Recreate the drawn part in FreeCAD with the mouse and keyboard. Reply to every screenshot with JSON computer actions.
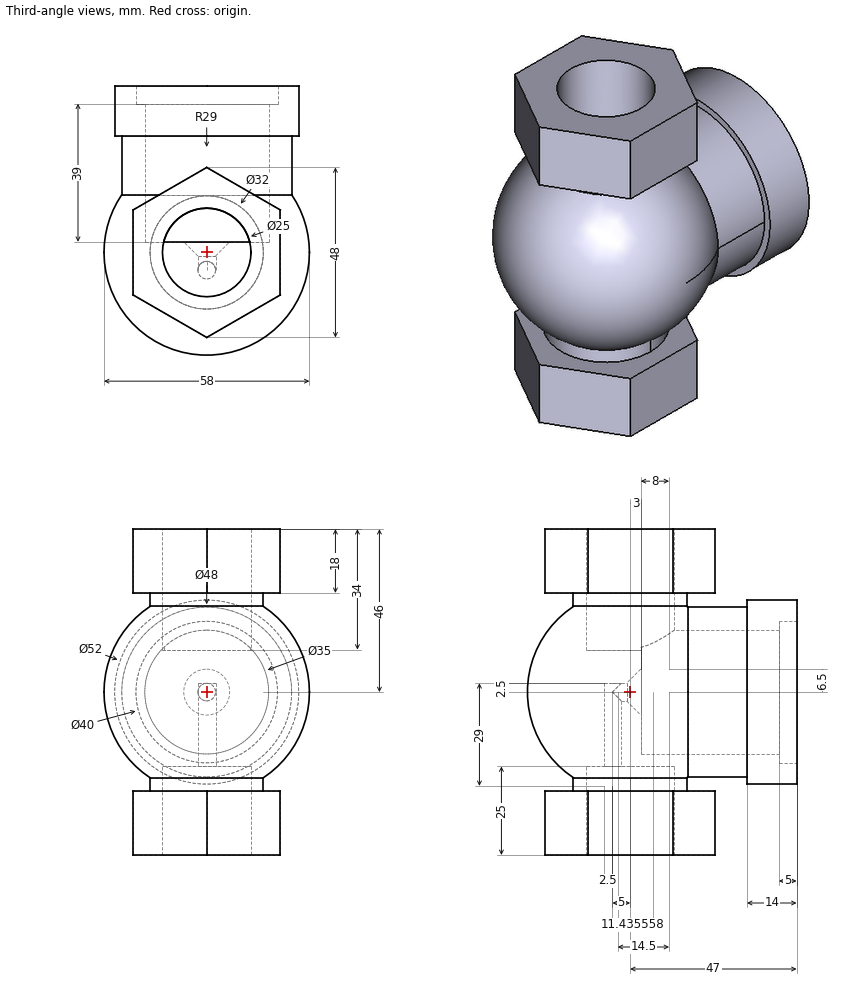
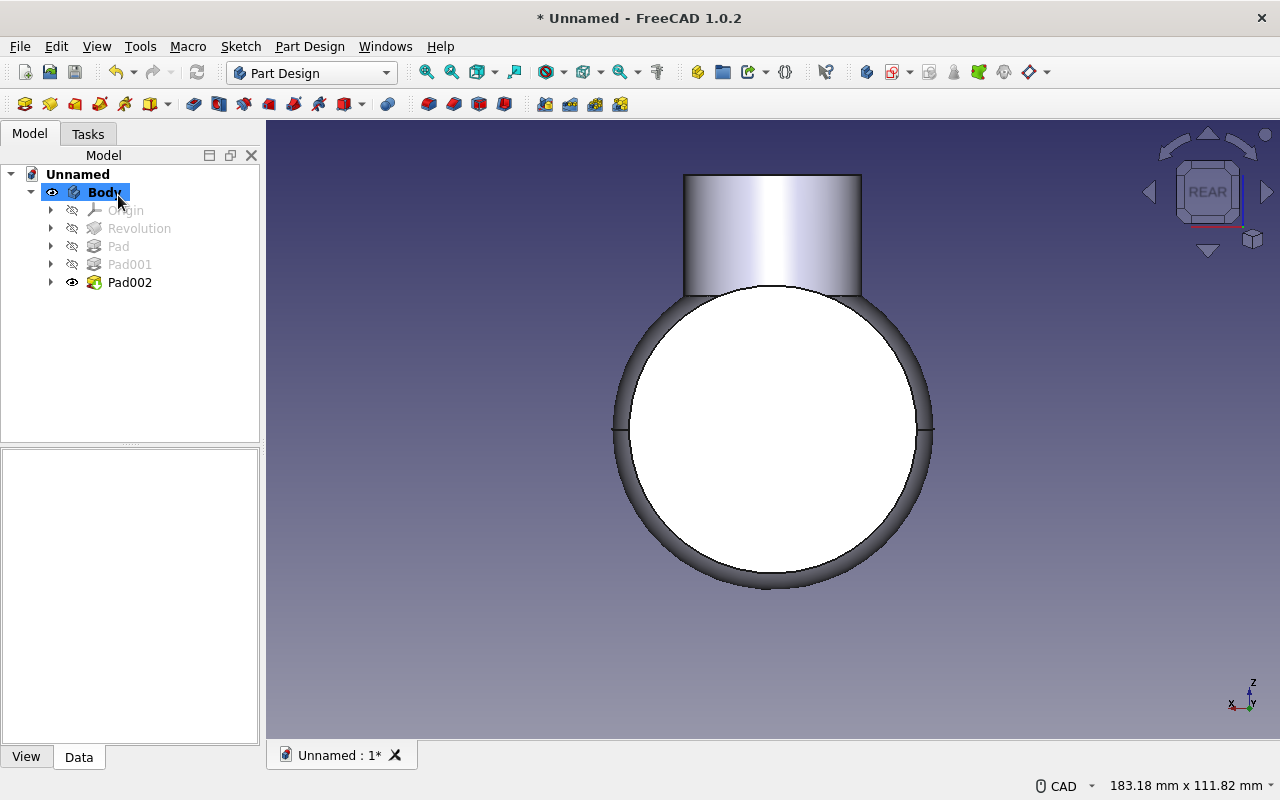
{"action": "left_click", "coordinate": [51, 210]}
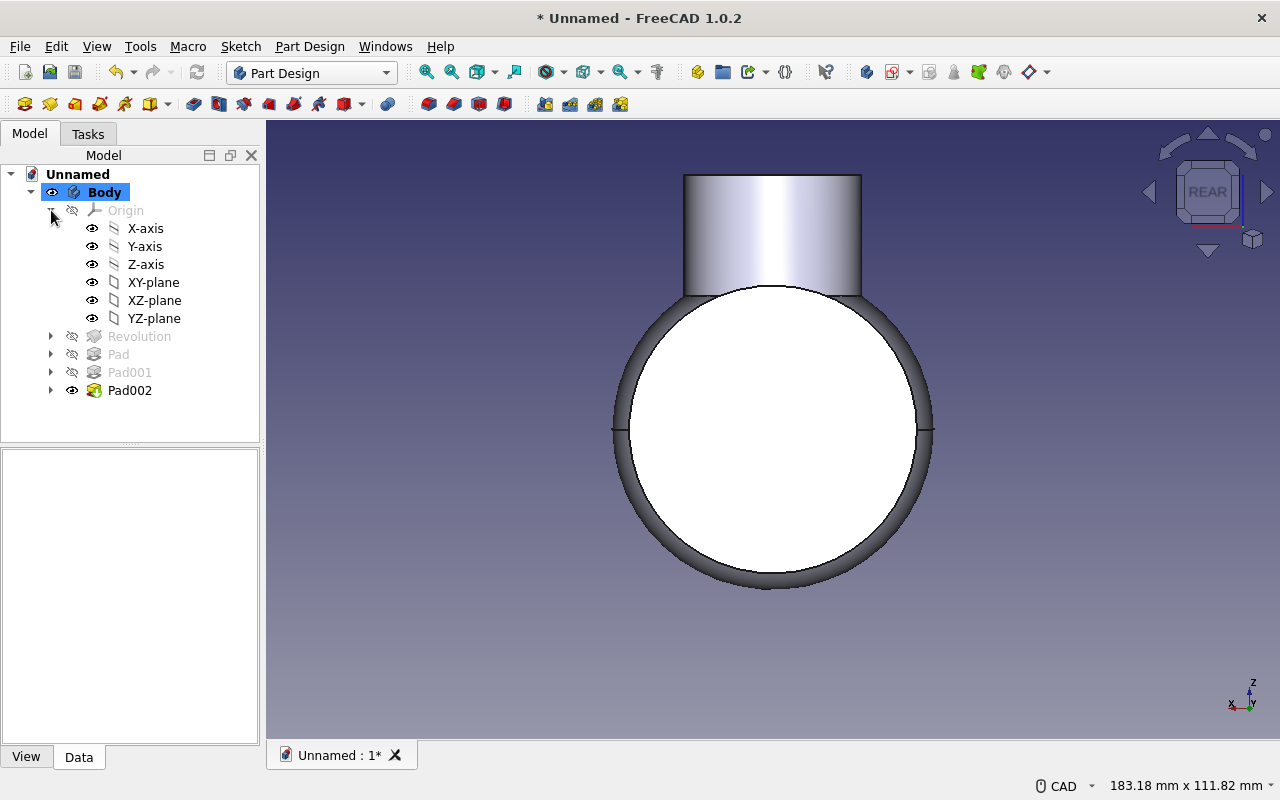
{"action": "left_click", "coordinate": [137, 282]}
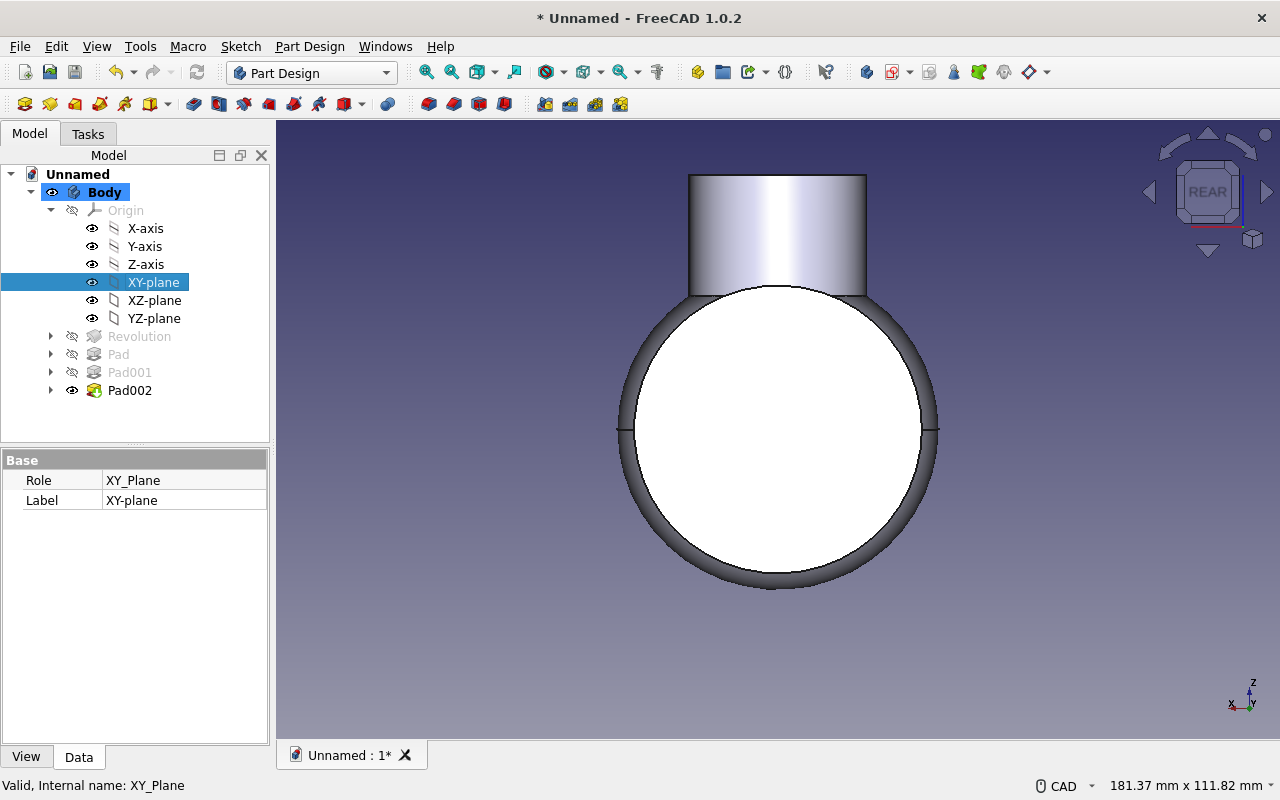
{"action": "left_click", "coordinate": [1028, 72]}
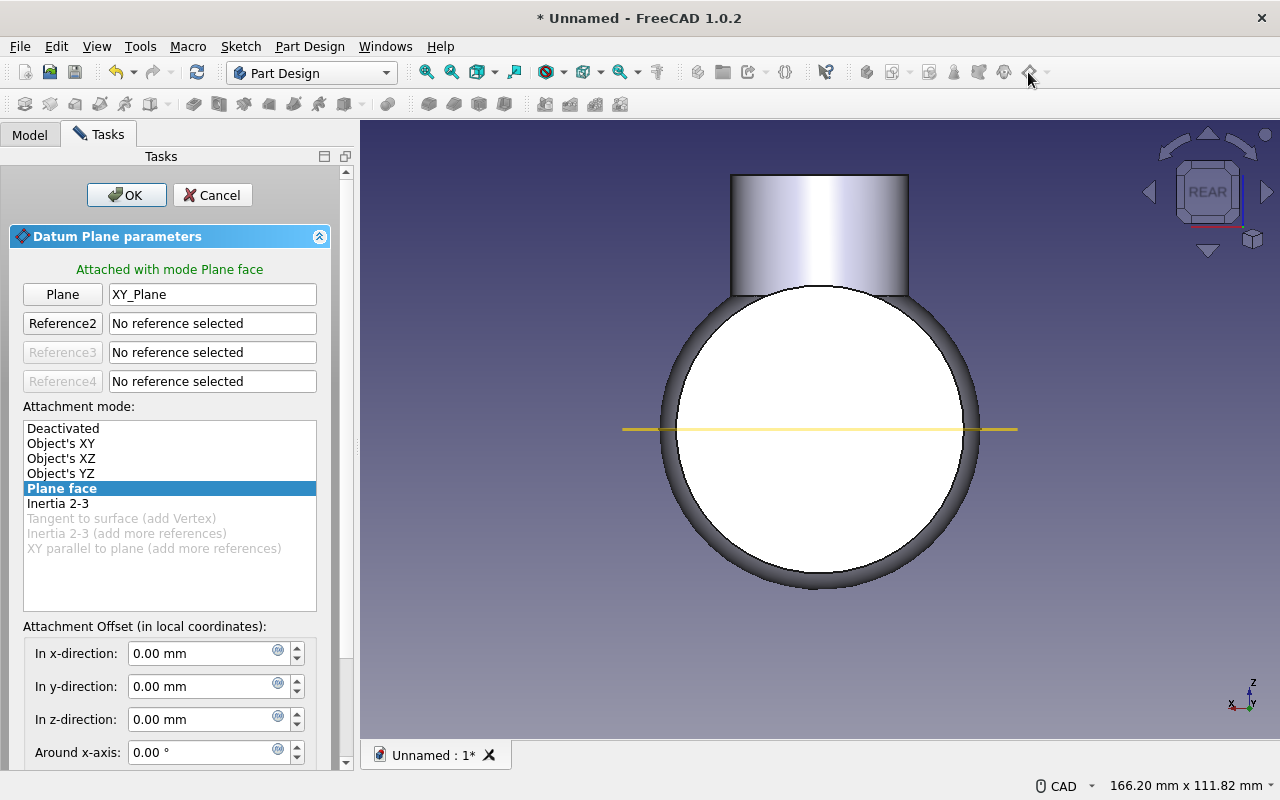
{"action": "triple_click", "coordinate": [210, 720]}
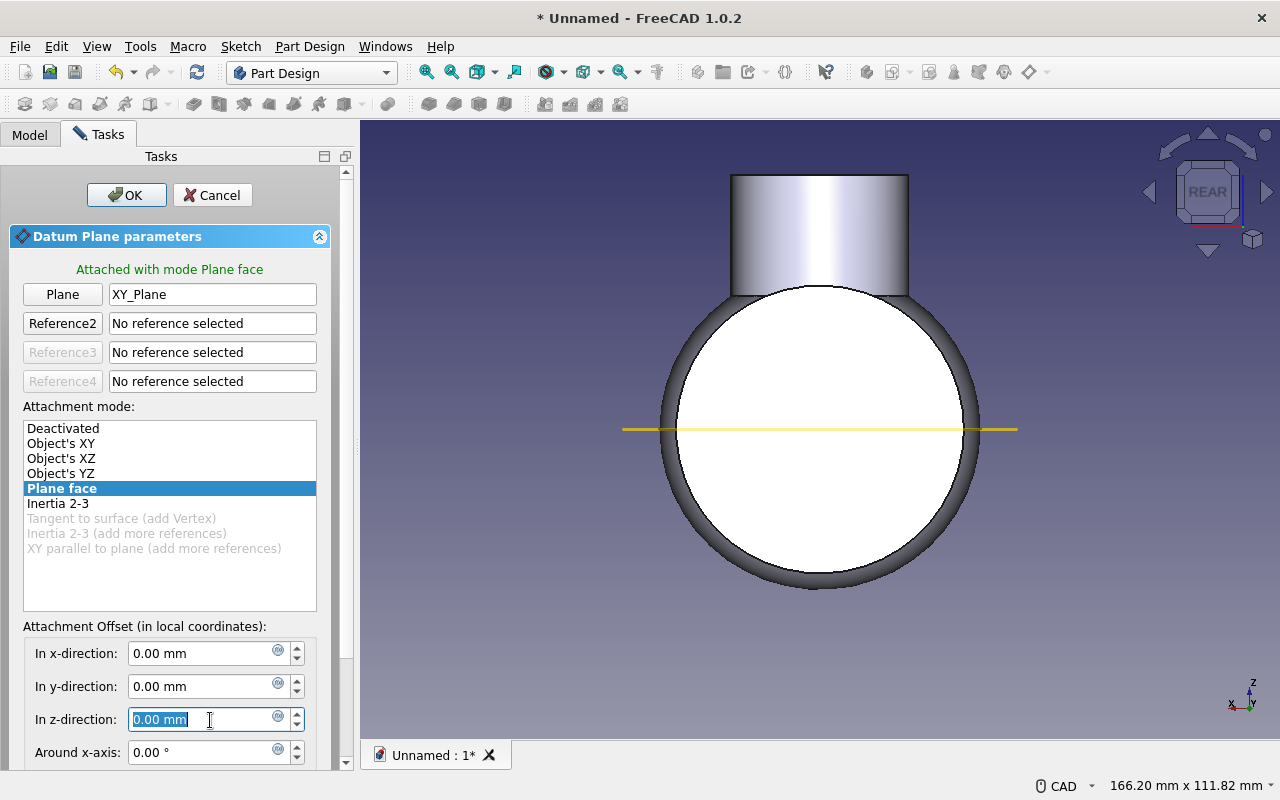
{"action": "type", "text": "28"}
{"action": "key", "text": "Tab"}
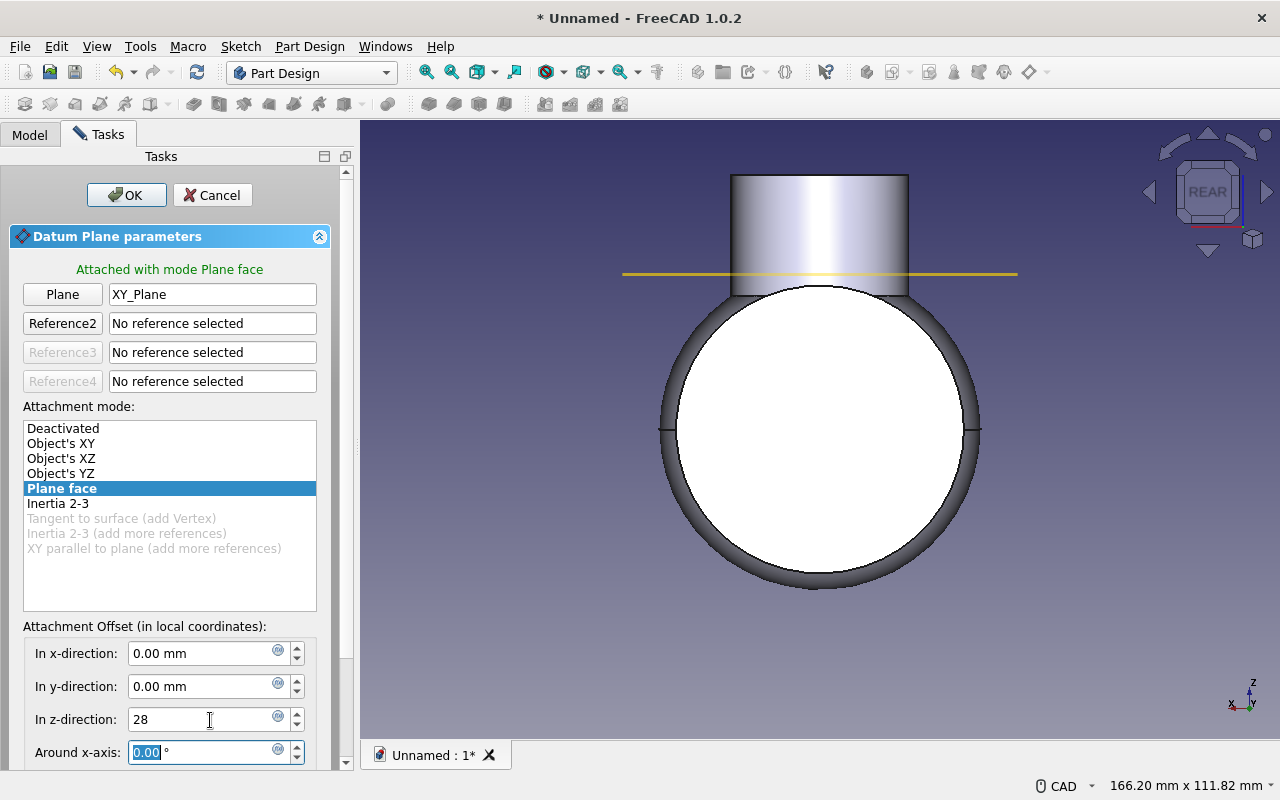
{"action": "left_click", "coordinate": [127, 195]}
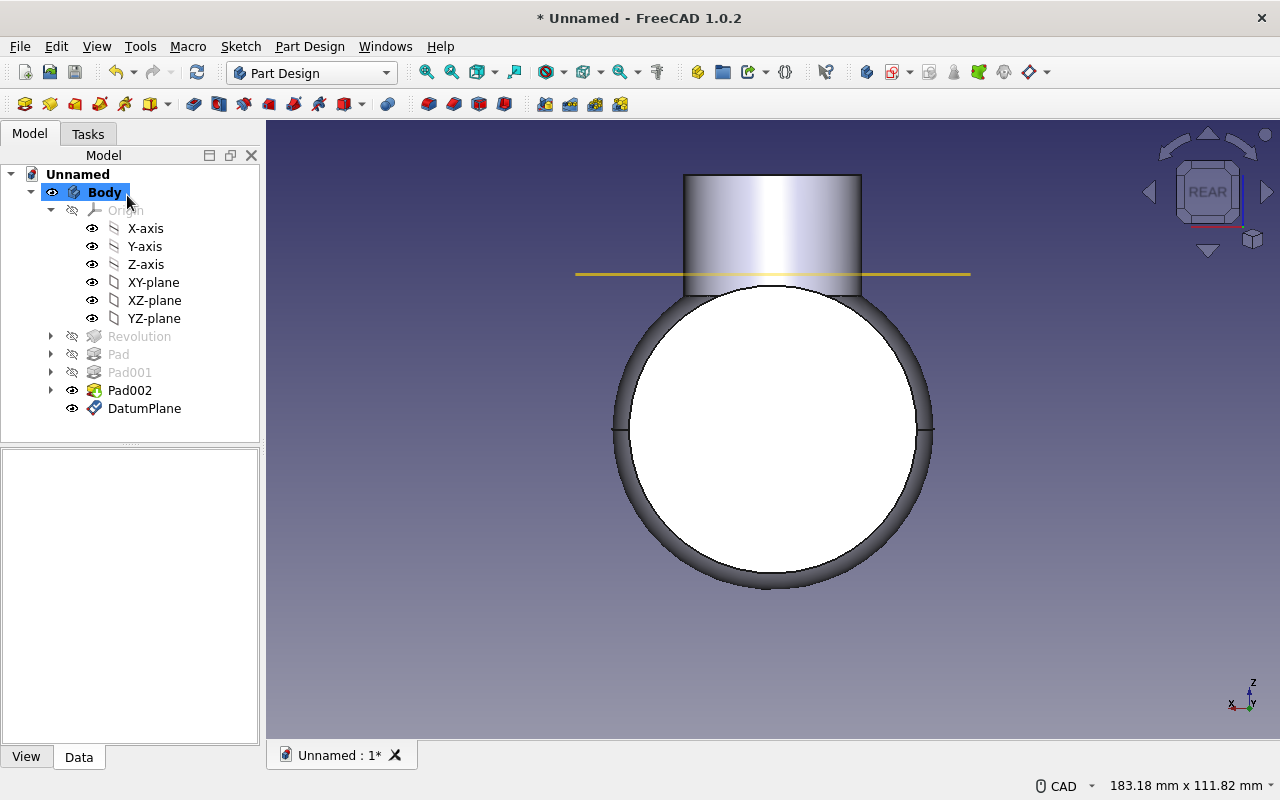
{"action": "left_click", "coordinate": [117, 408]}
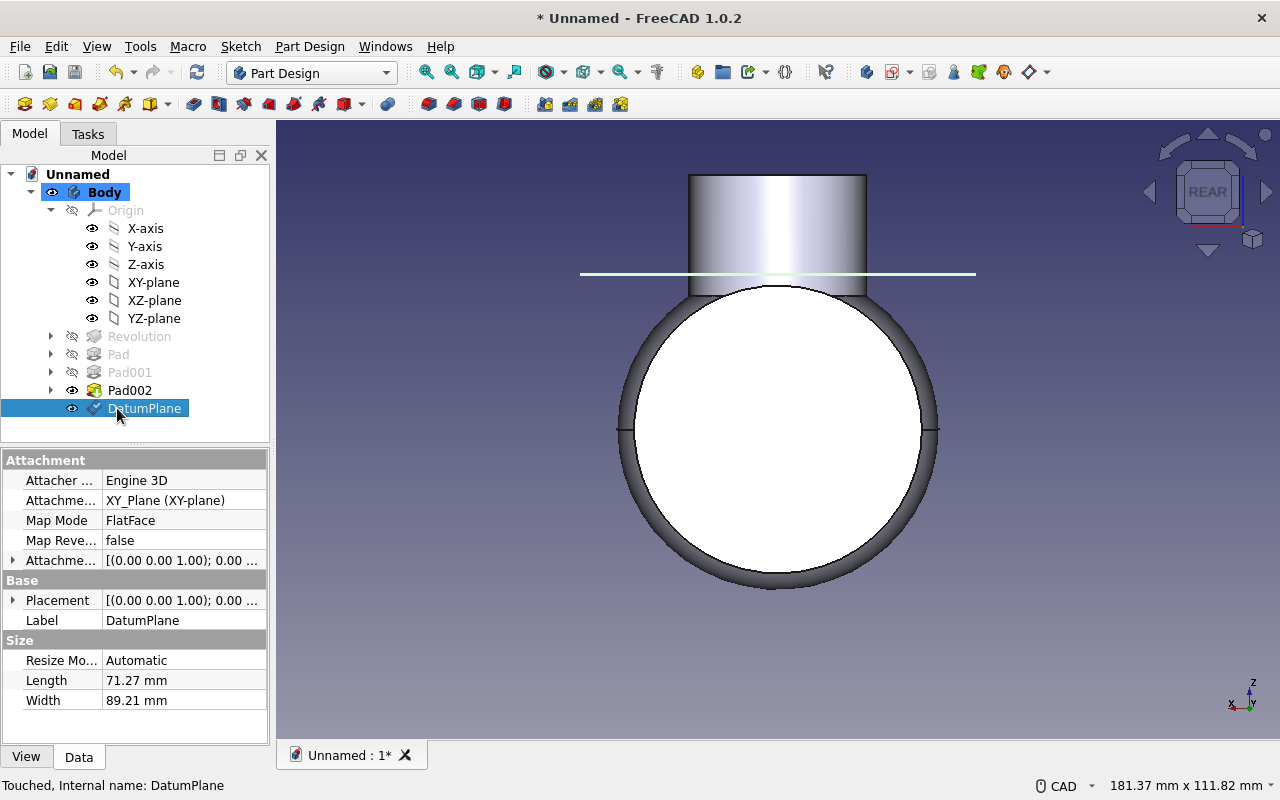
{"action": "left_click", "coordinate": [892, 72]}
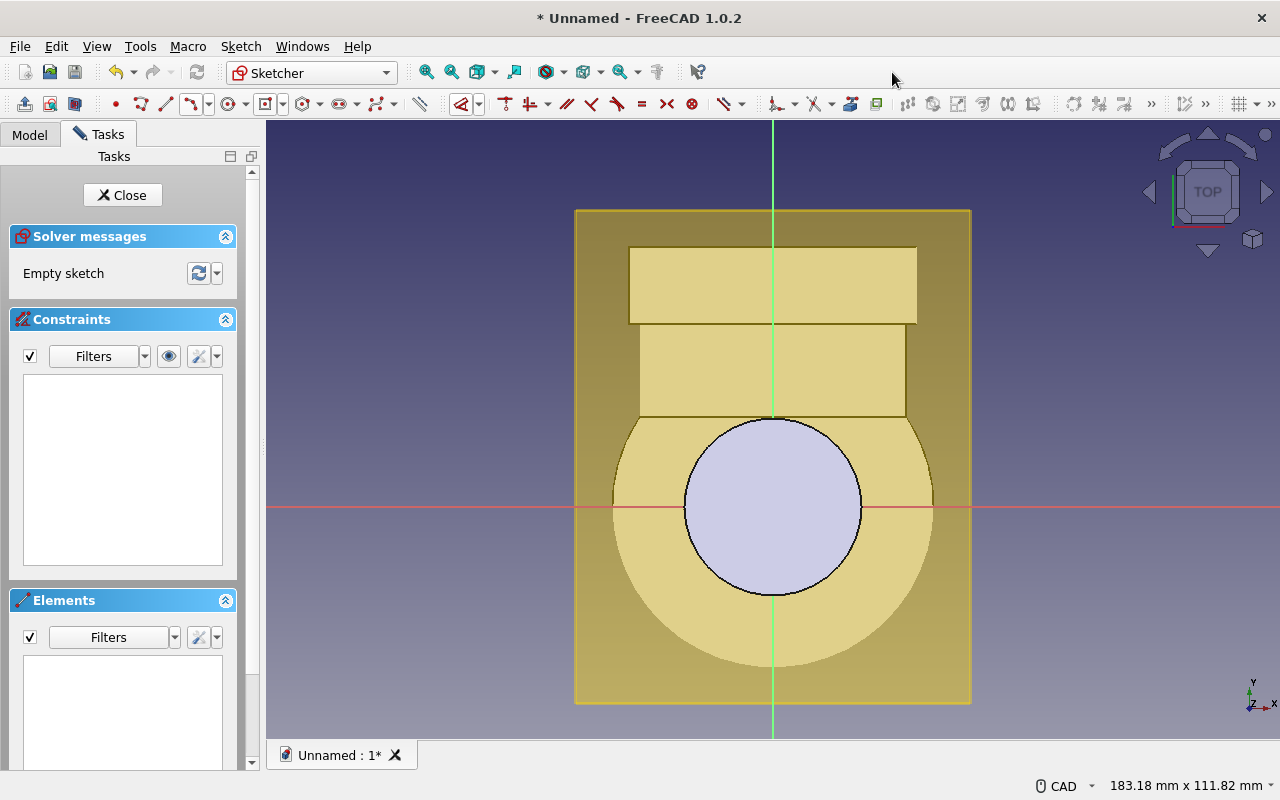
{"action": "left_click", "coordinate": [75, 104]}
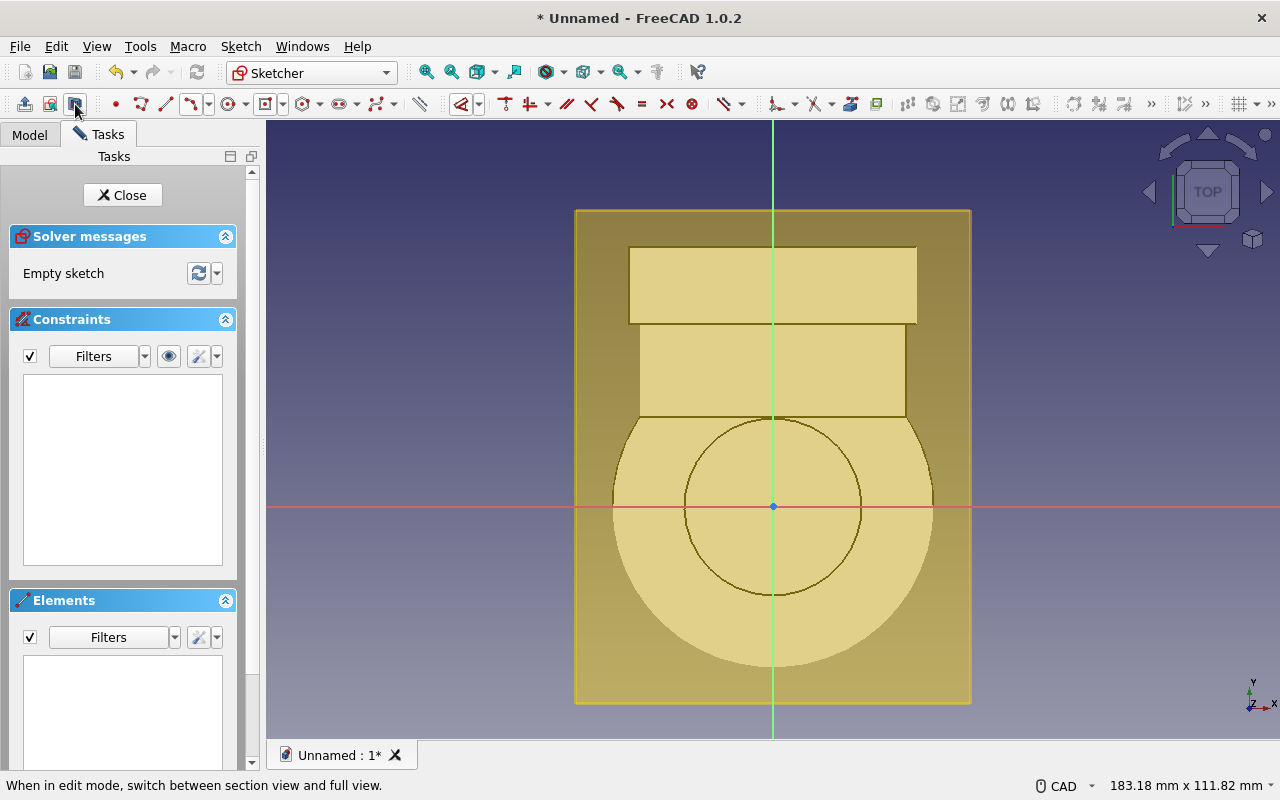
{"action": "scroll", "coordinate": [912, 665], "scroll_direction": "up", "scroll_amount": 2}